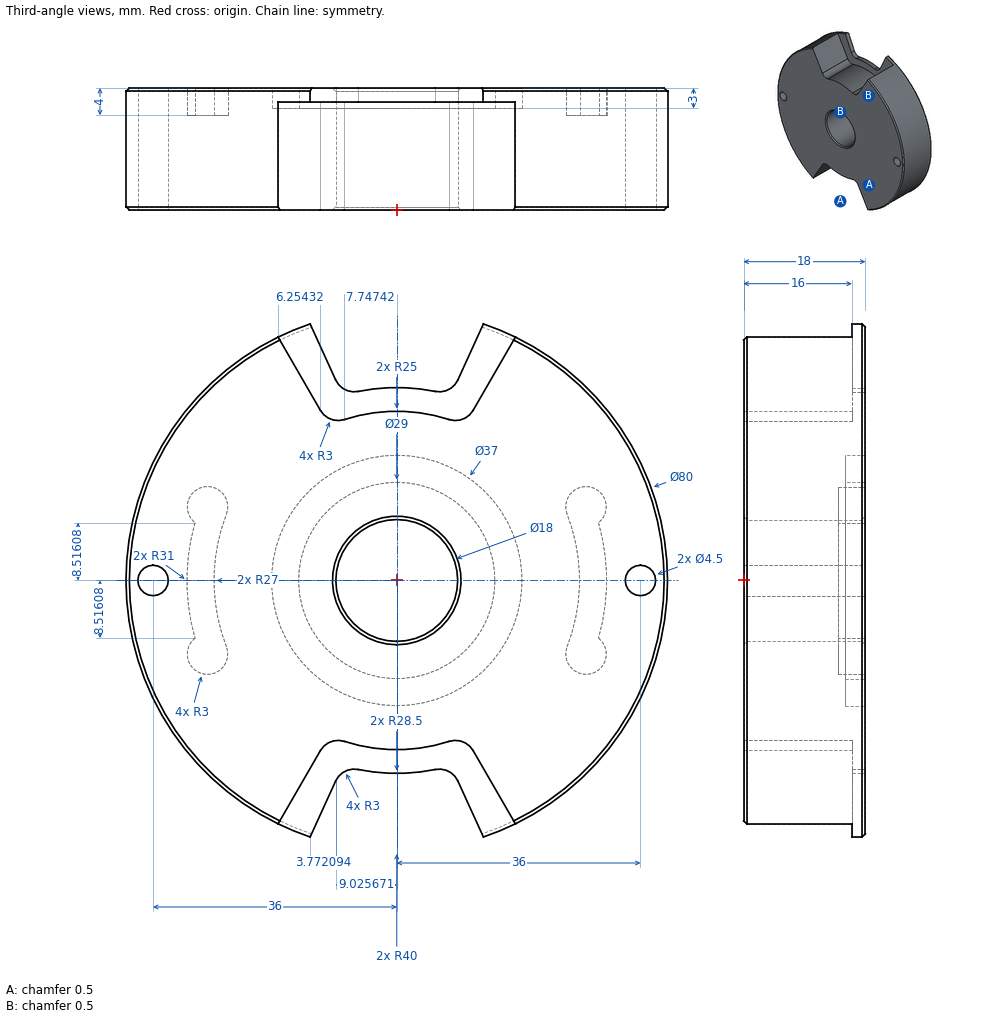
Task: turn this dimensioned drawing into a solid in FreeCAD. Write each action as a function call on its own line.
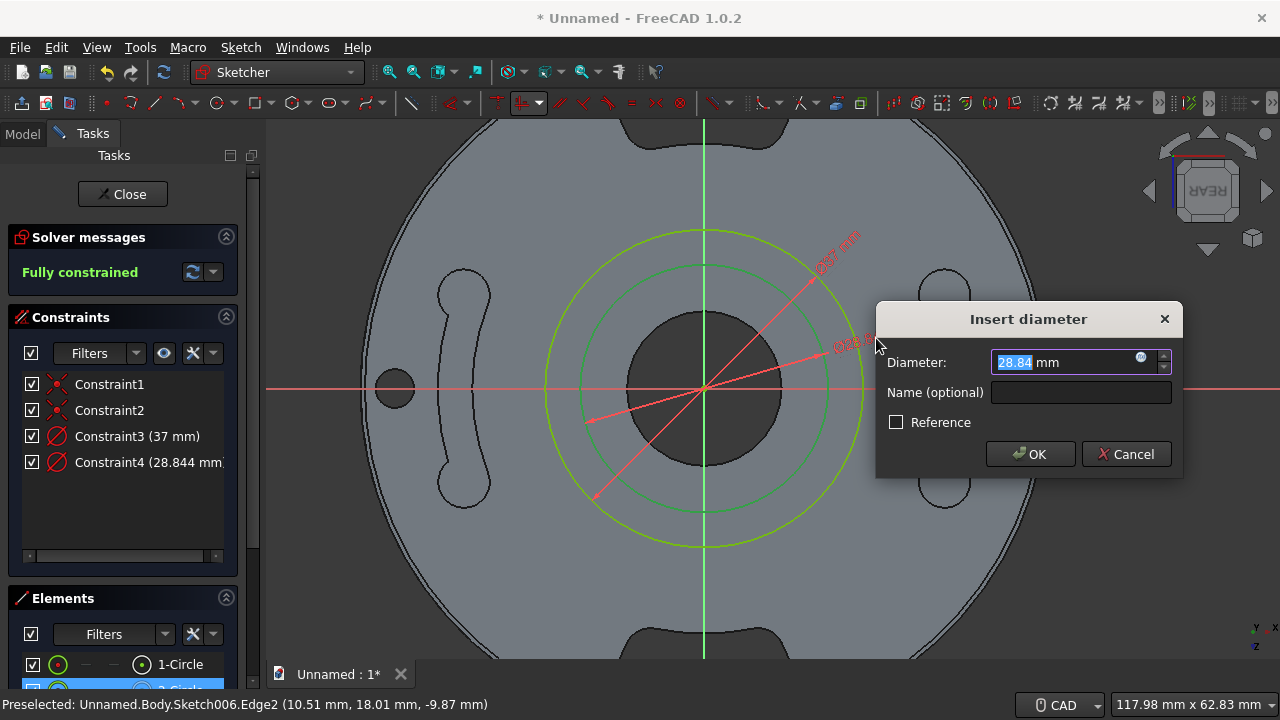
text(29)
key(Return)
key(Escape)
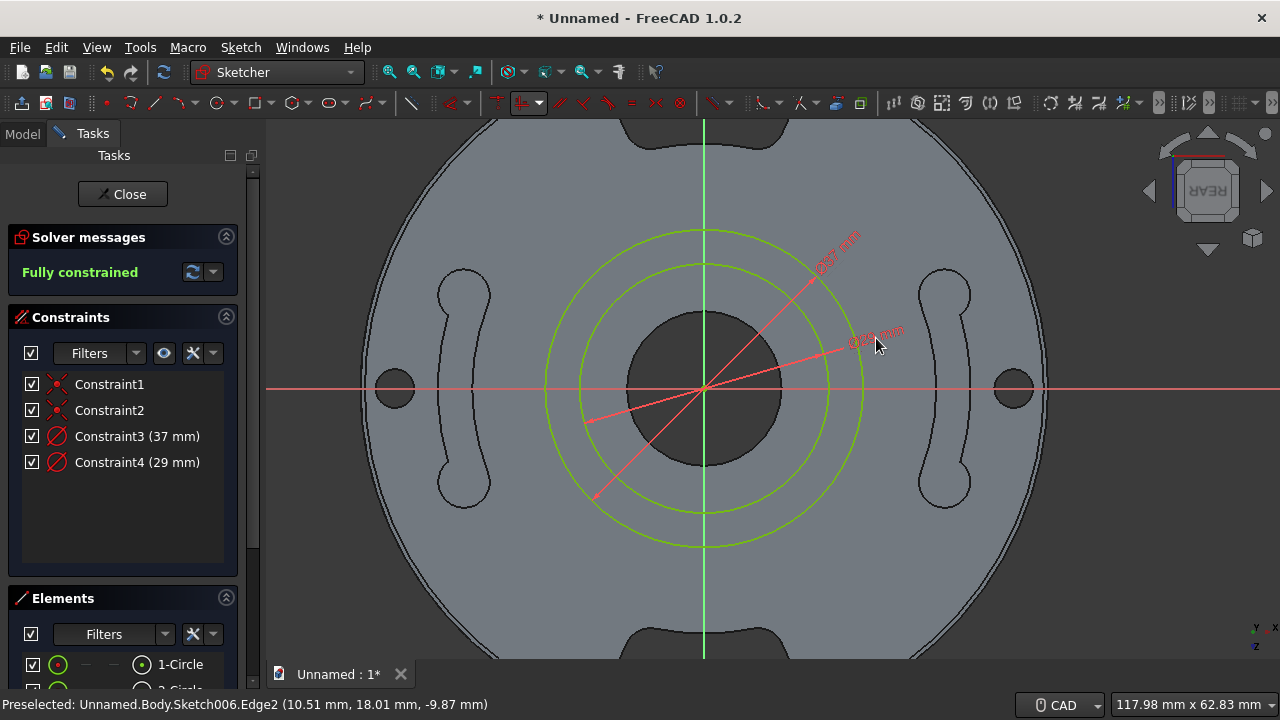
click(123, 194)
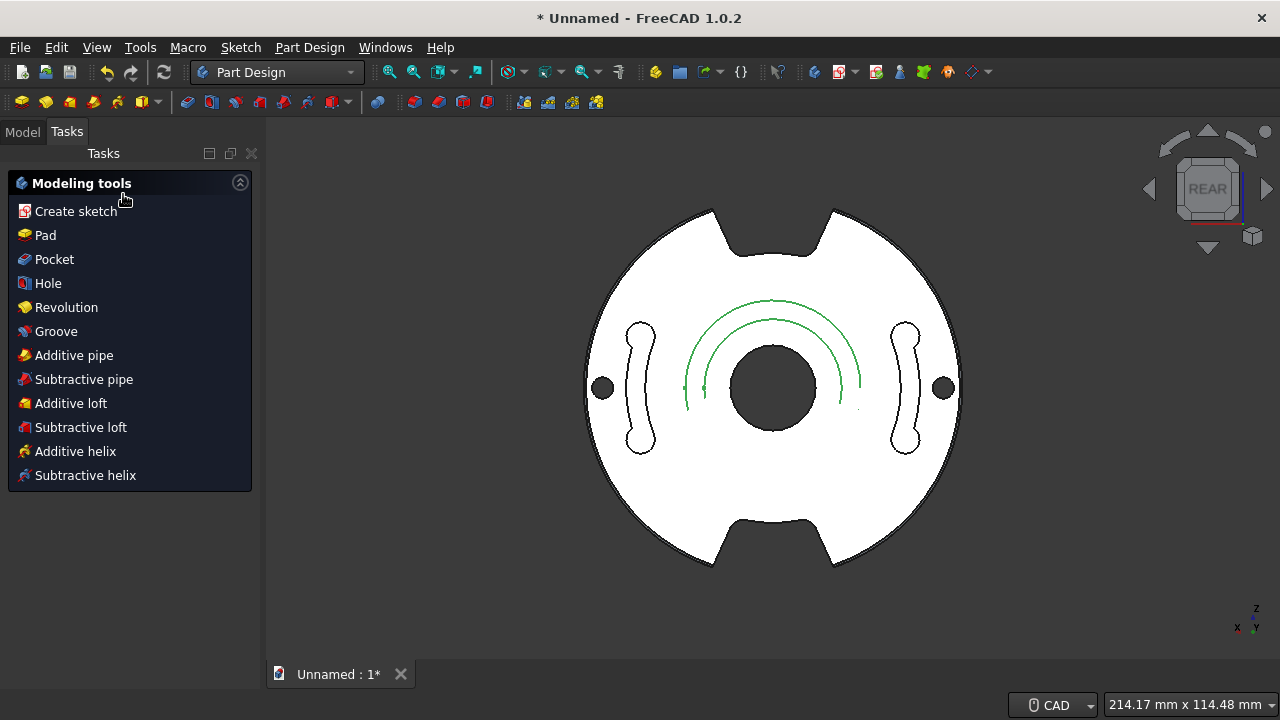
click(188, 102)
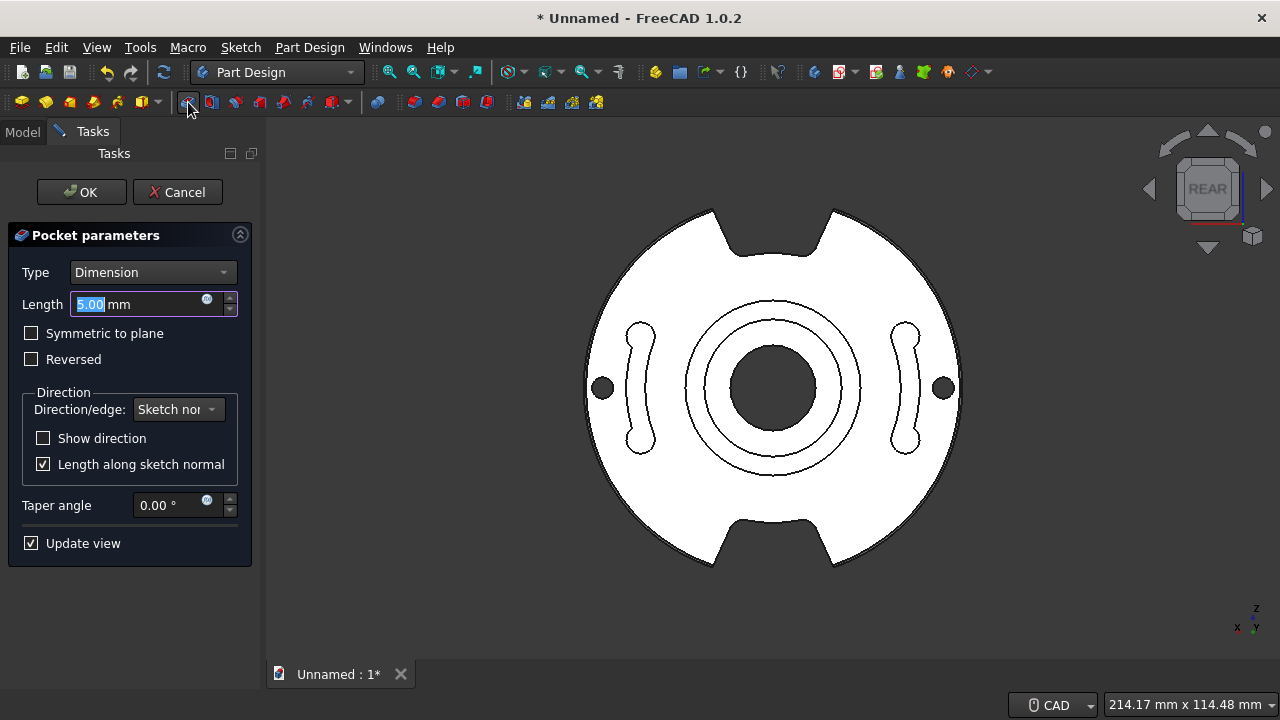
text(3)
key(Tab)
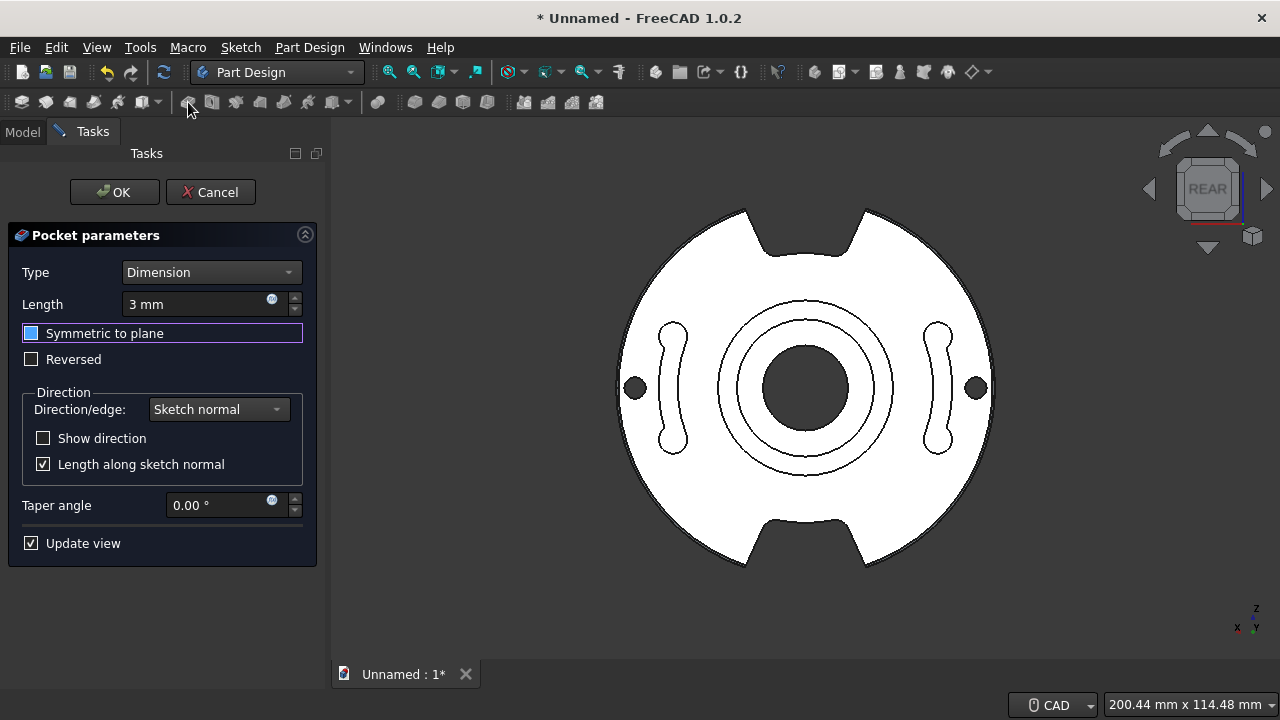
click(115, 192)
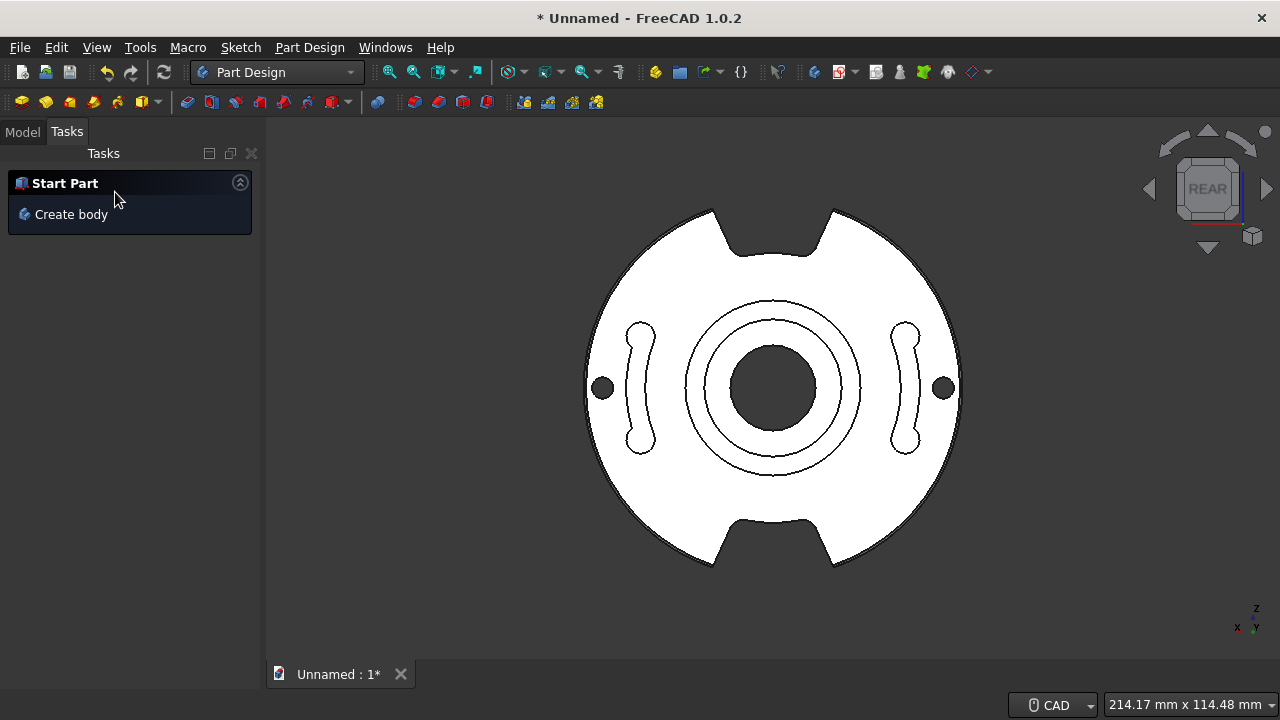
click(807, 362)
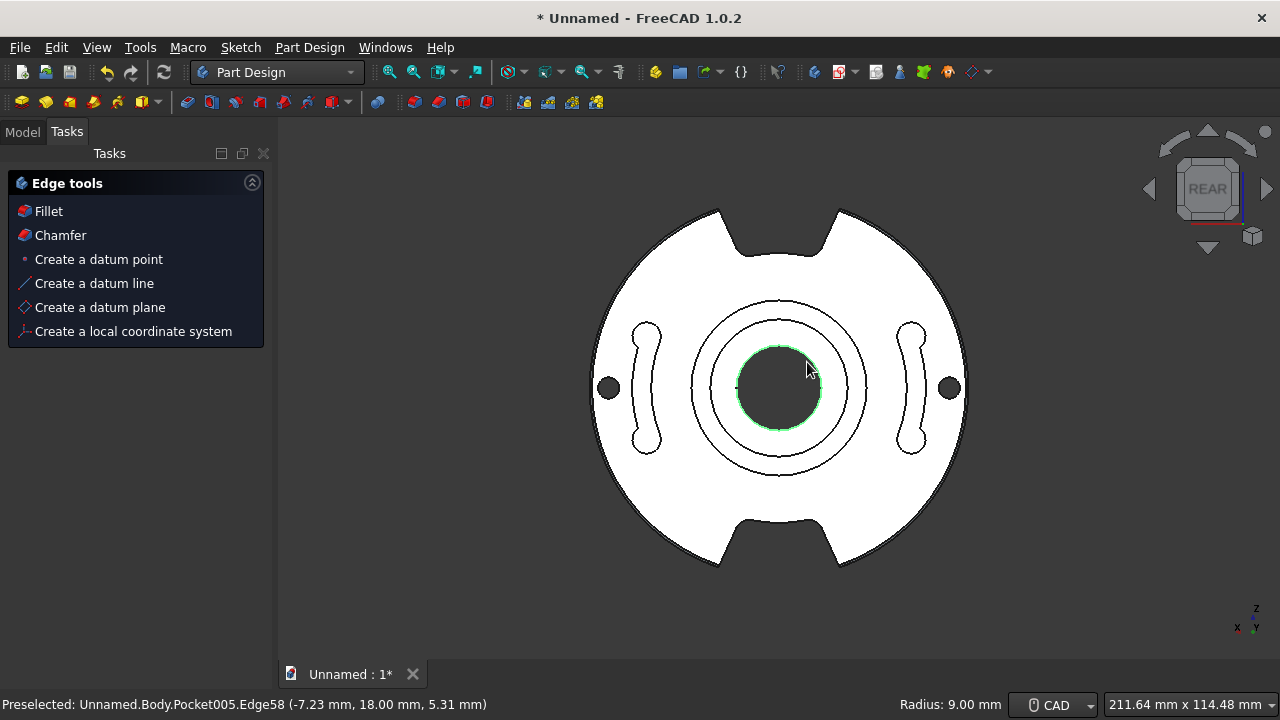
key(0)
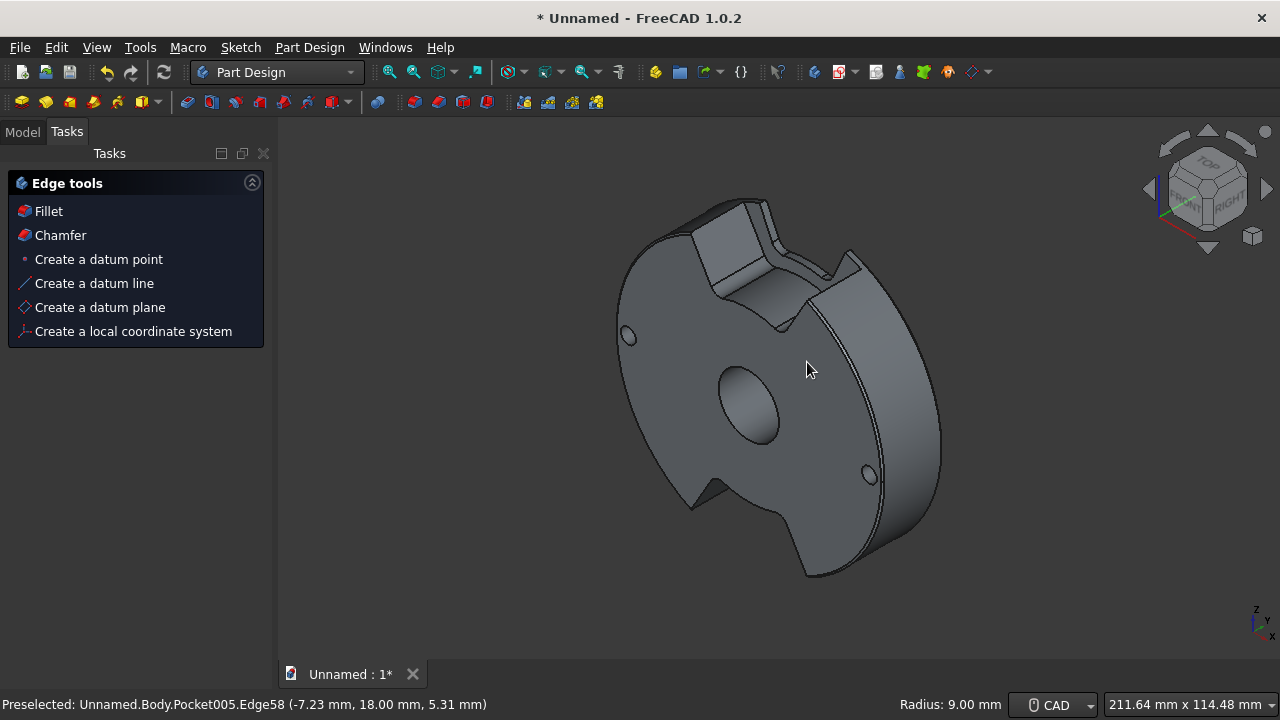
click(719, 387, ctrl)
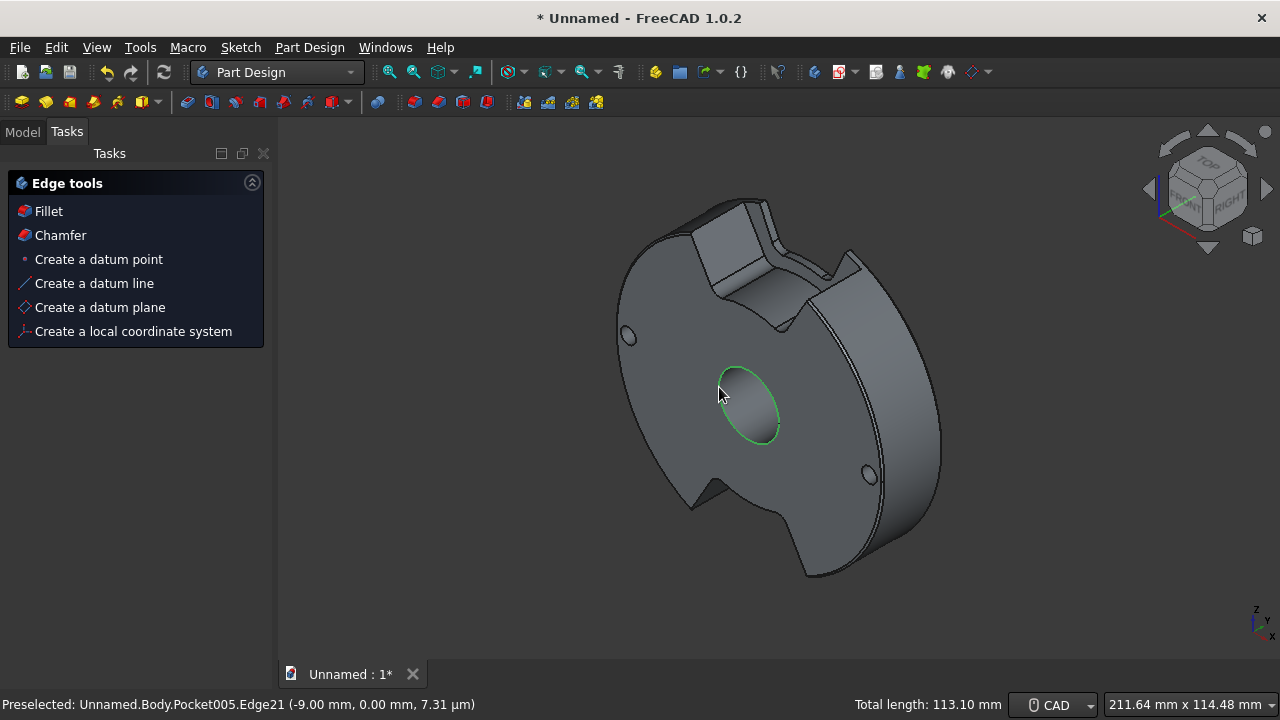
click(440, 102)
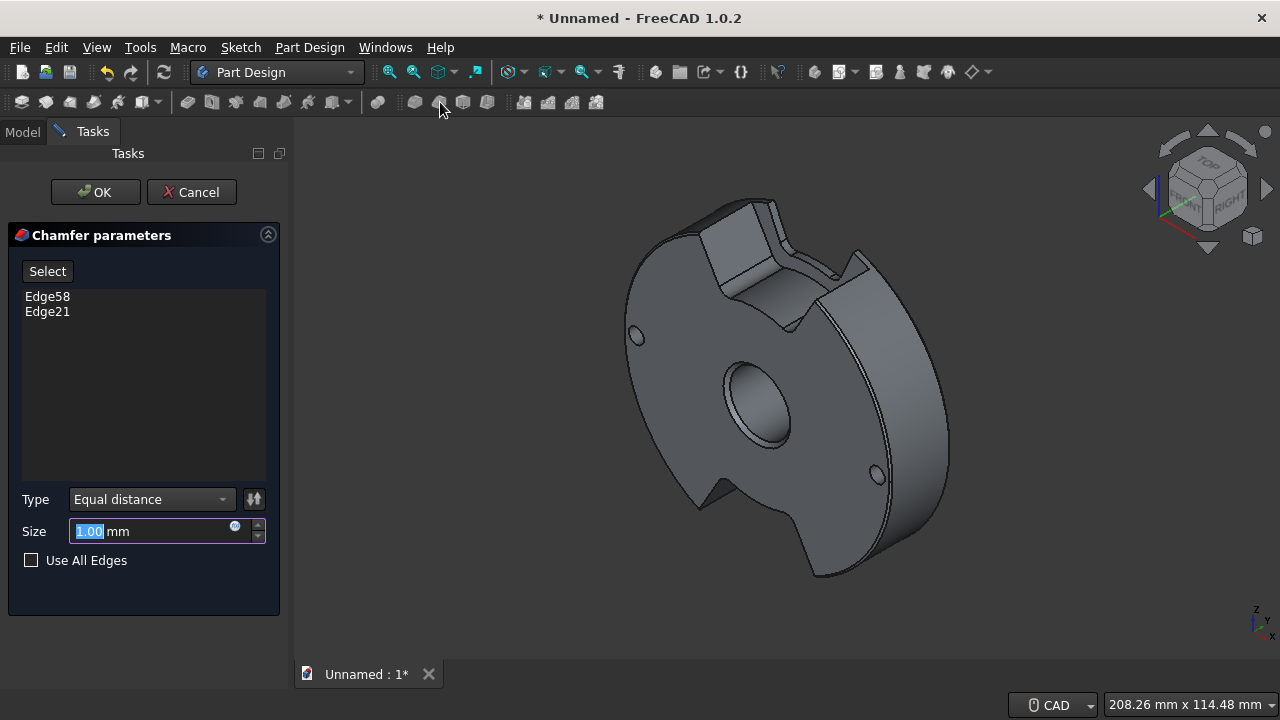
text(0.5)
key(Tab)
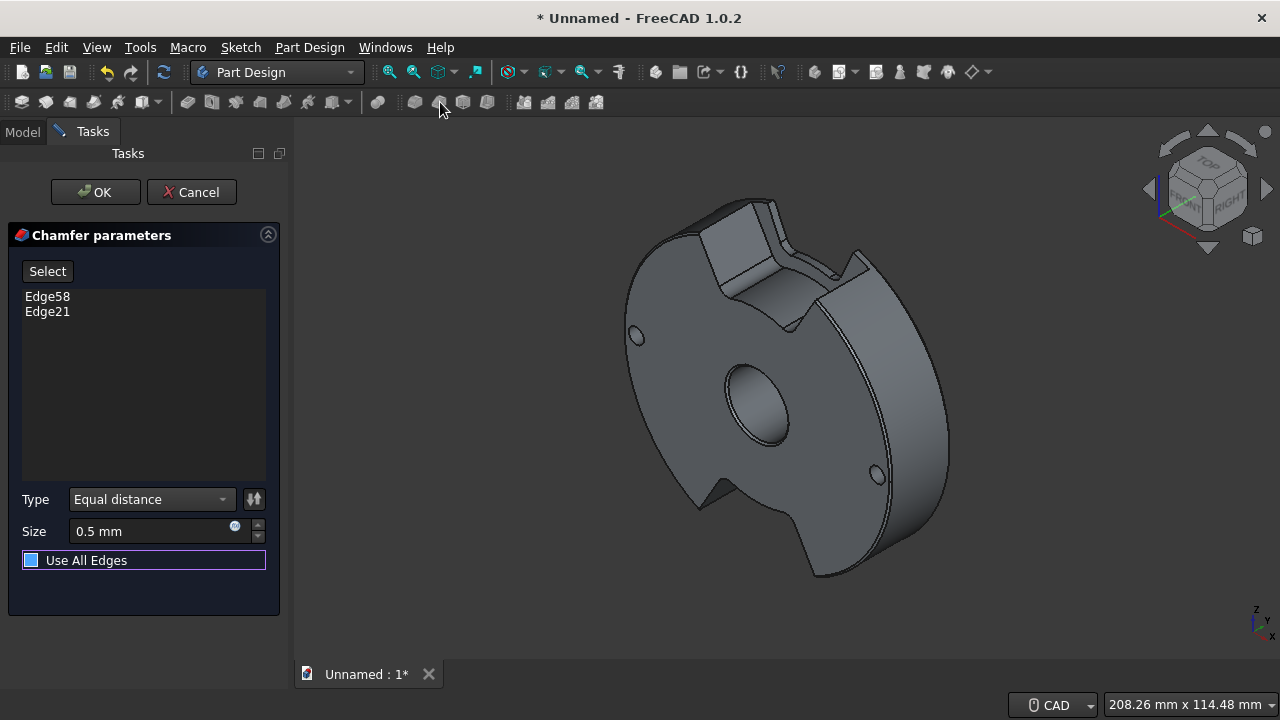
click(96, 192)